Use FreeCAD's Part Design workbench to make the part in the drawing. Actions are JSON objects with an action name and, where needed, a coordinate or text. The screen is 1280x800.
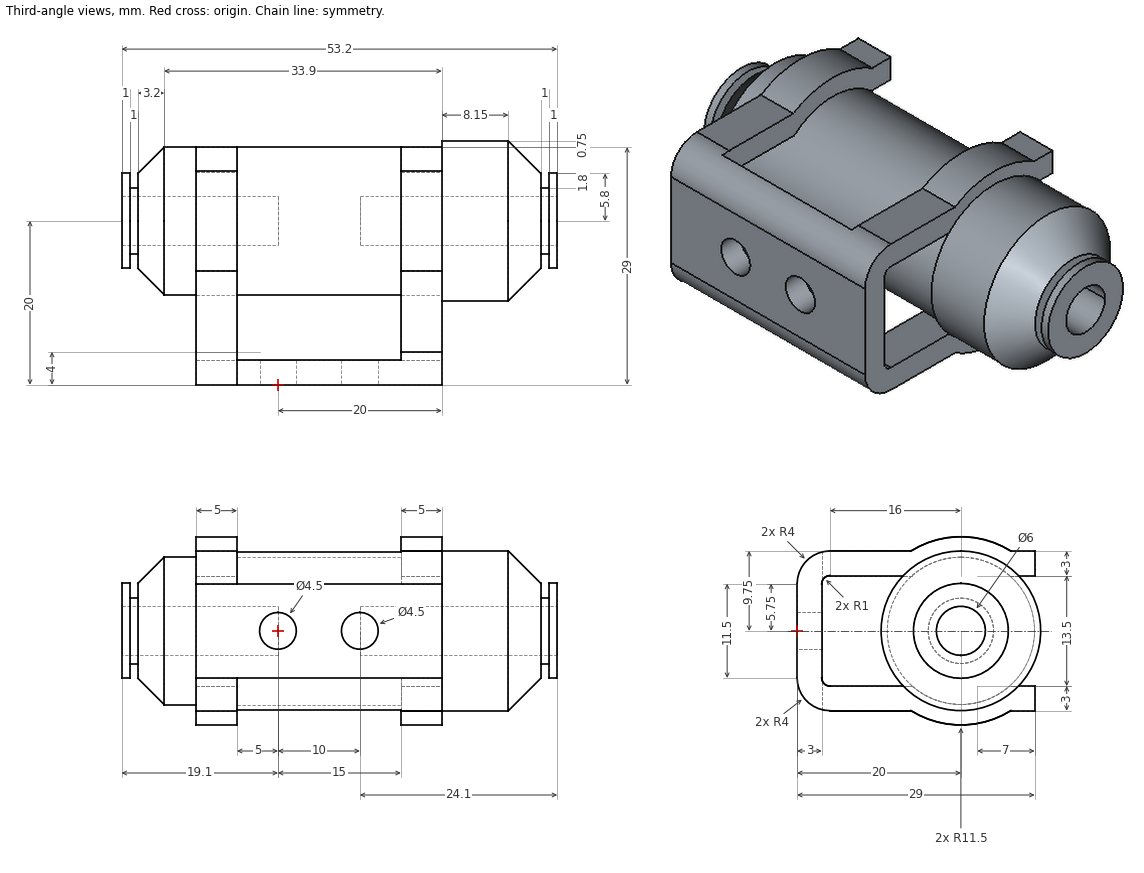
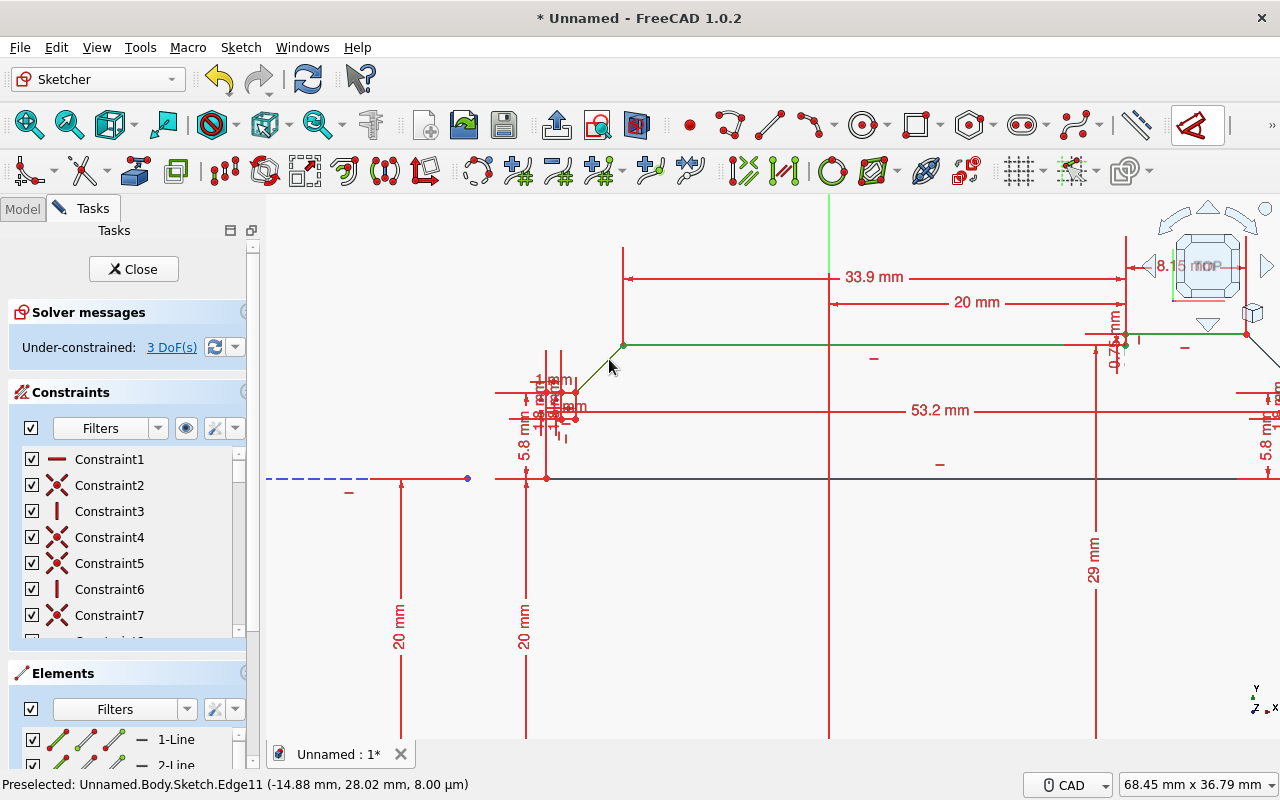
{"action": "key", "text": "l"}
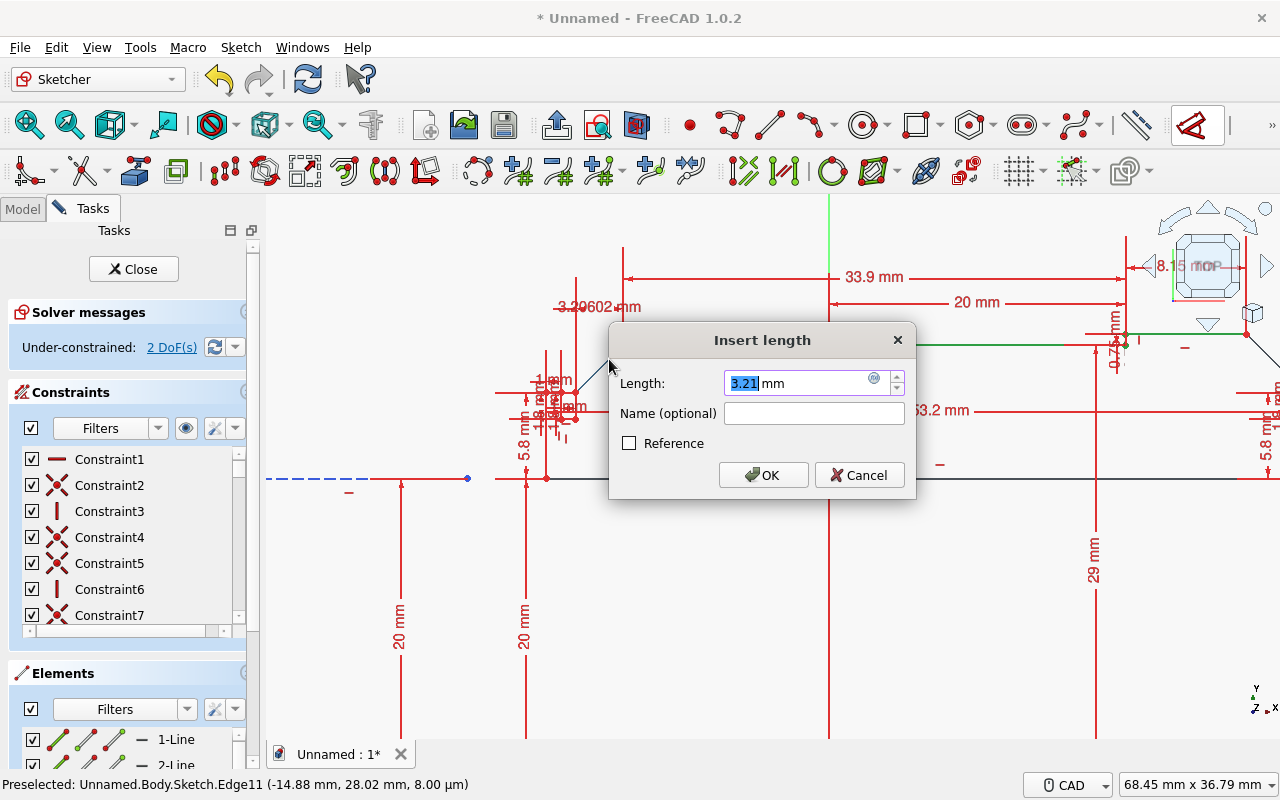
{"action": "type", "text": "3.2"}
{"action": "key", "text": "Return"}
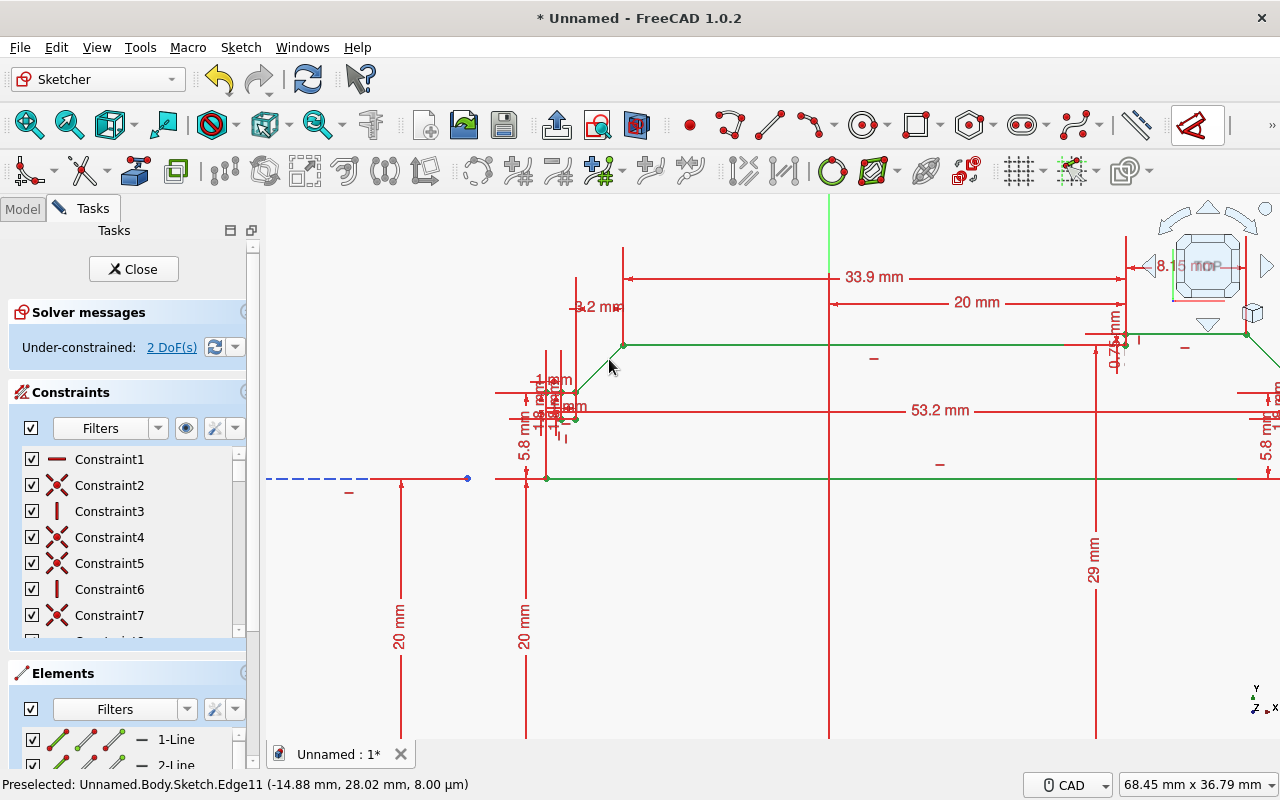
{"action": "left_click", "coordinate": [134, 269]}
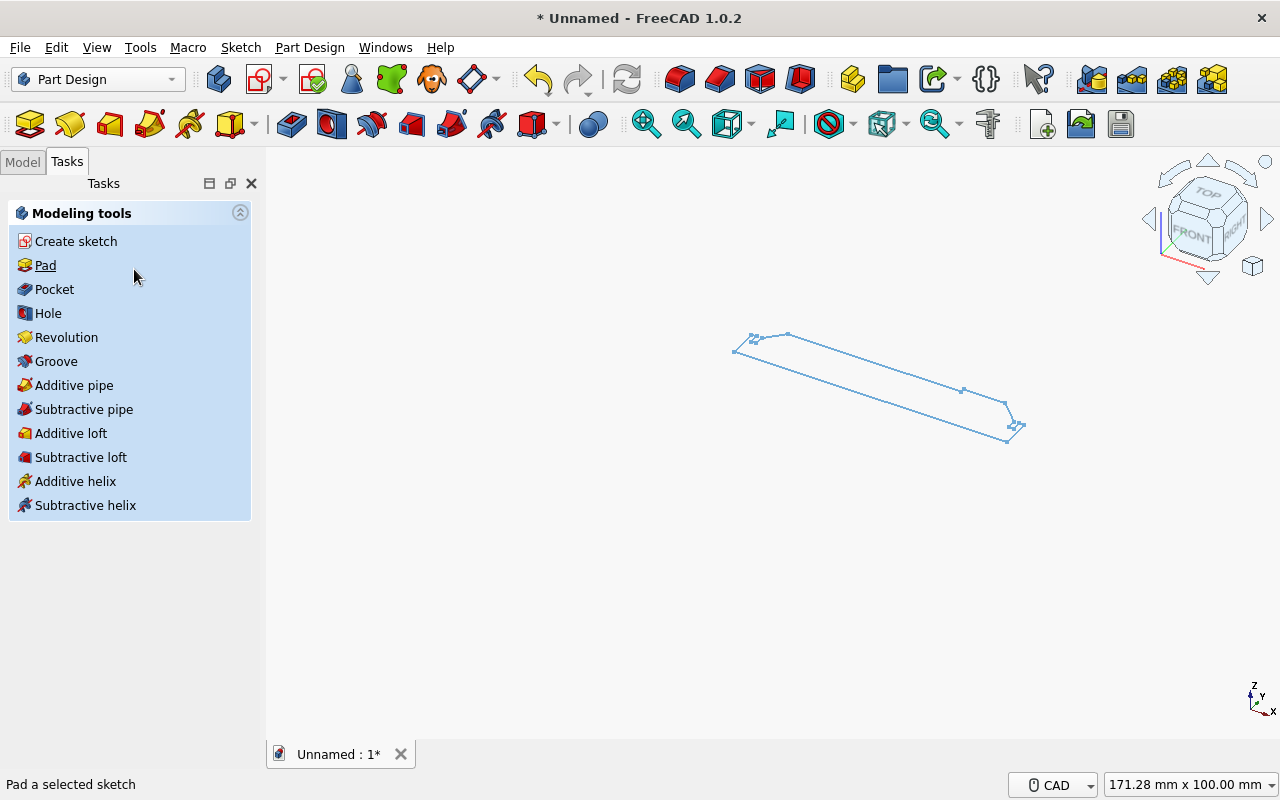
{"action": "left_click", "coordinate": [70, 124]}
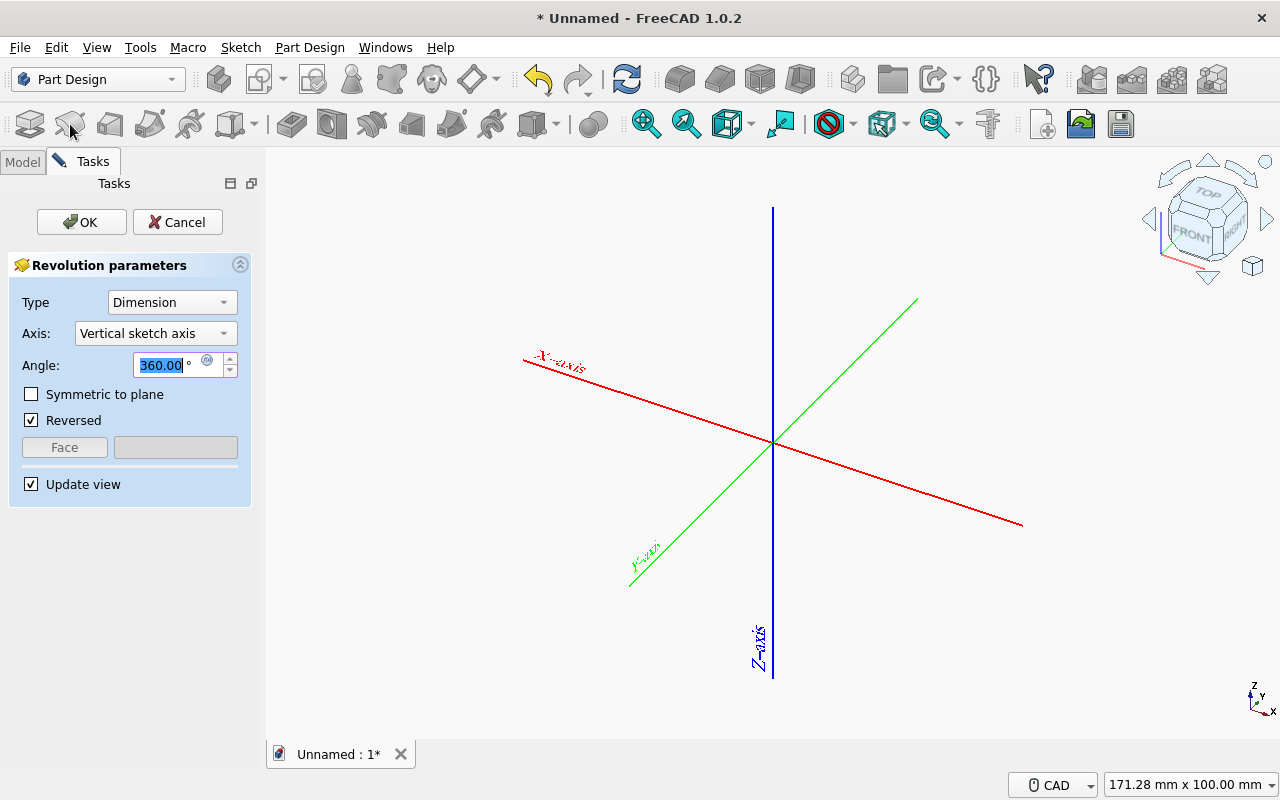
{"action": "left_click", "coordinate": [156, 334]}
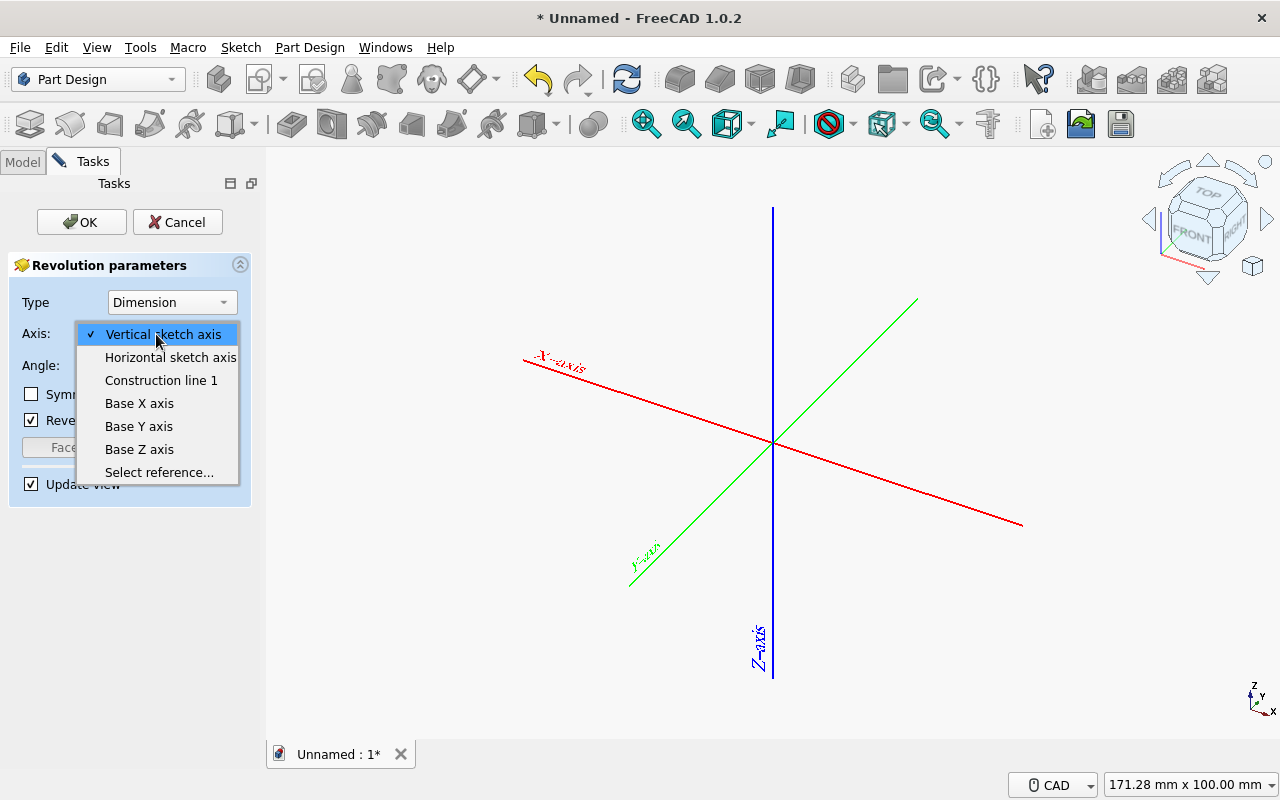
{"action": "left_click", "coordinate": [156, 380]}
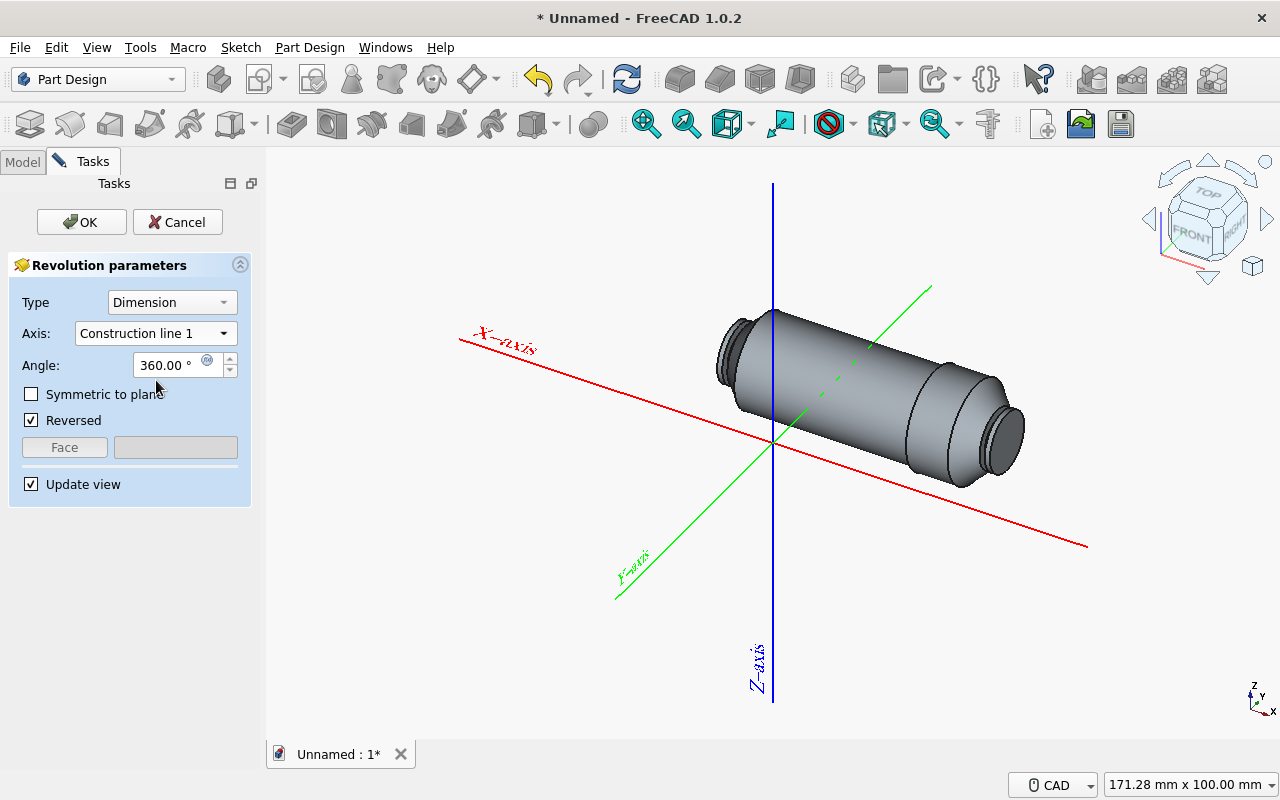
{"action": "left_click", "coordinate": [82, 222]}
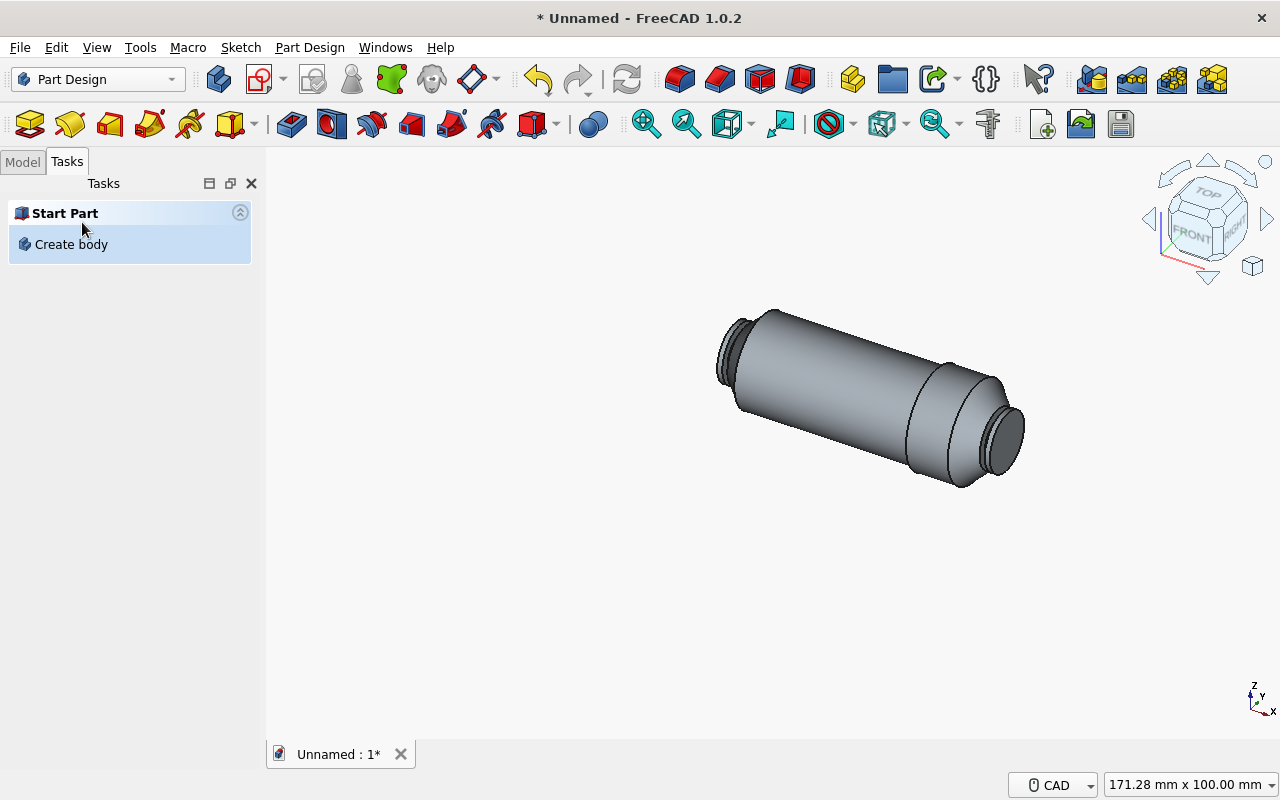
{"action": "left_click", "coordinate": [648, 124]}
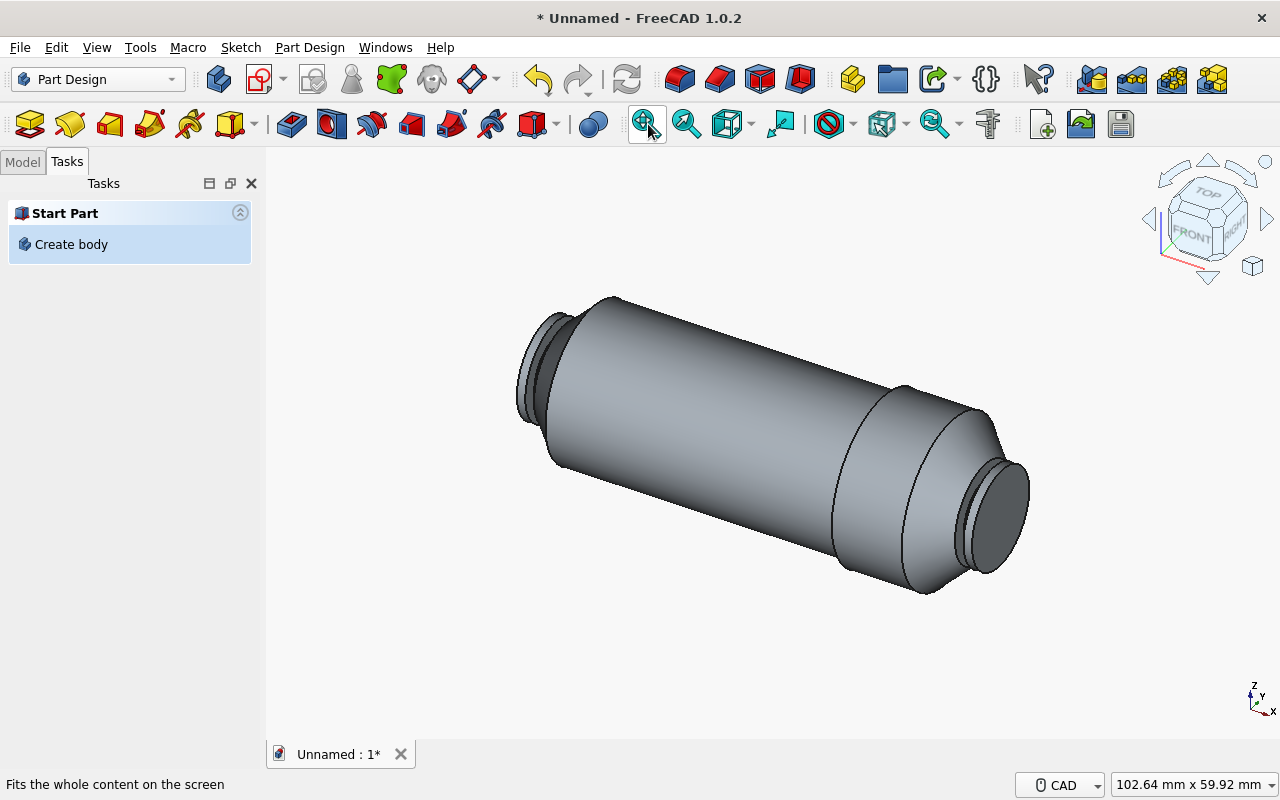
{"action": "left_click", "coordinate": [23, 161]}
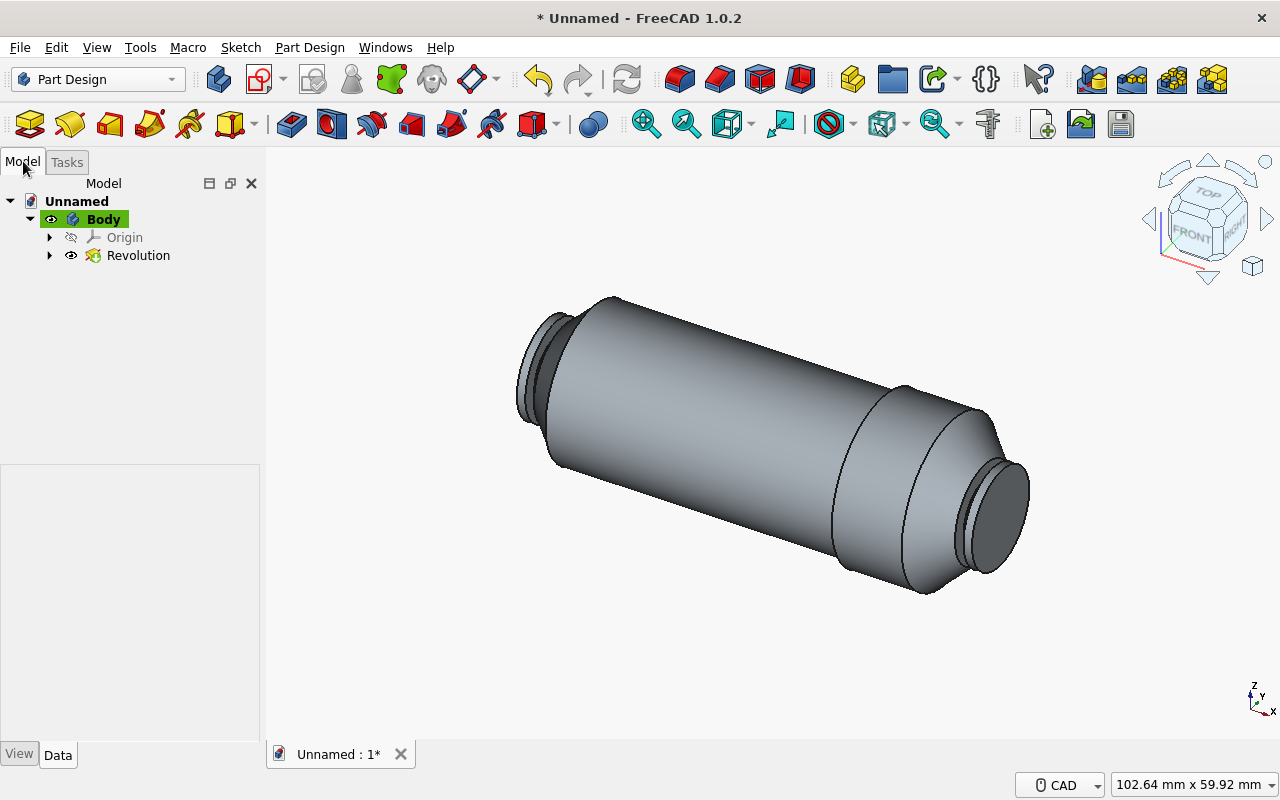
{"action": "left_click", "coordinate": [50, 237]}